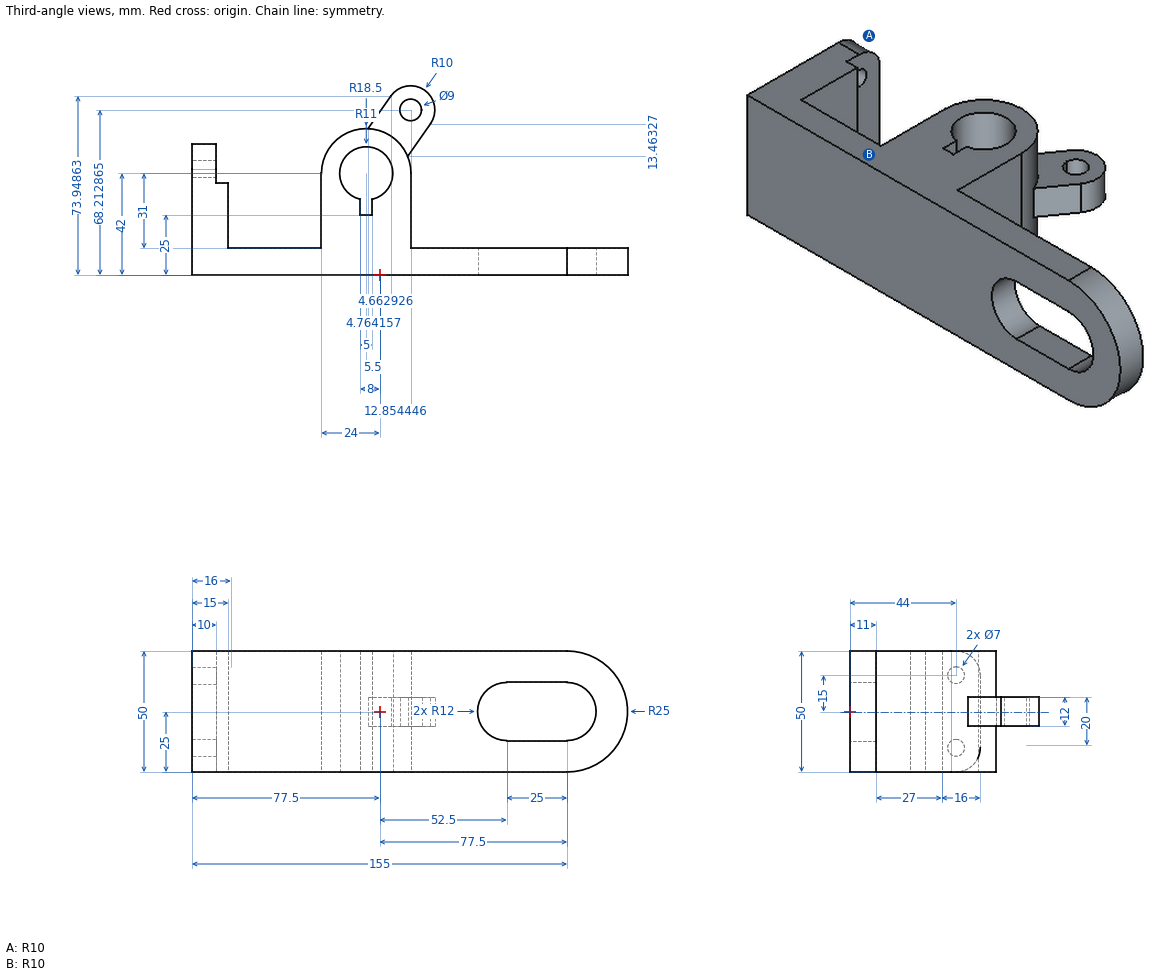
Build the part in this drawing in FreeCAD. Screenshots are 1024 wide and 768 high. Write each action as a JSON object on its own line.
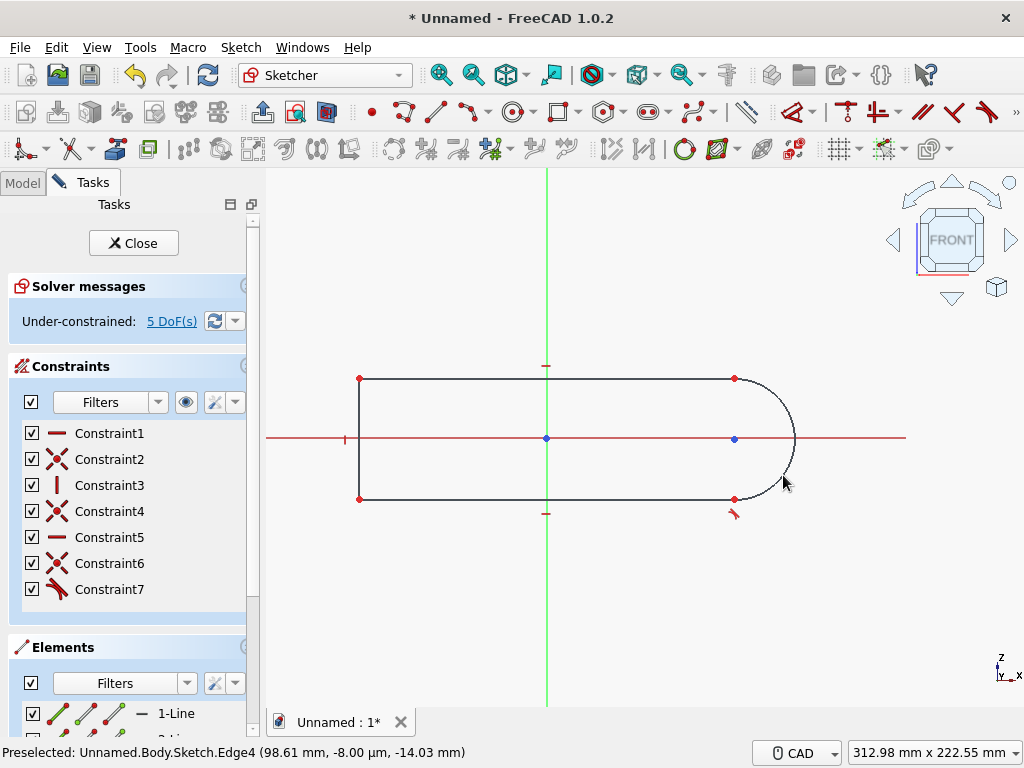
{"action": "left_click", "coordinate": [472, 379]}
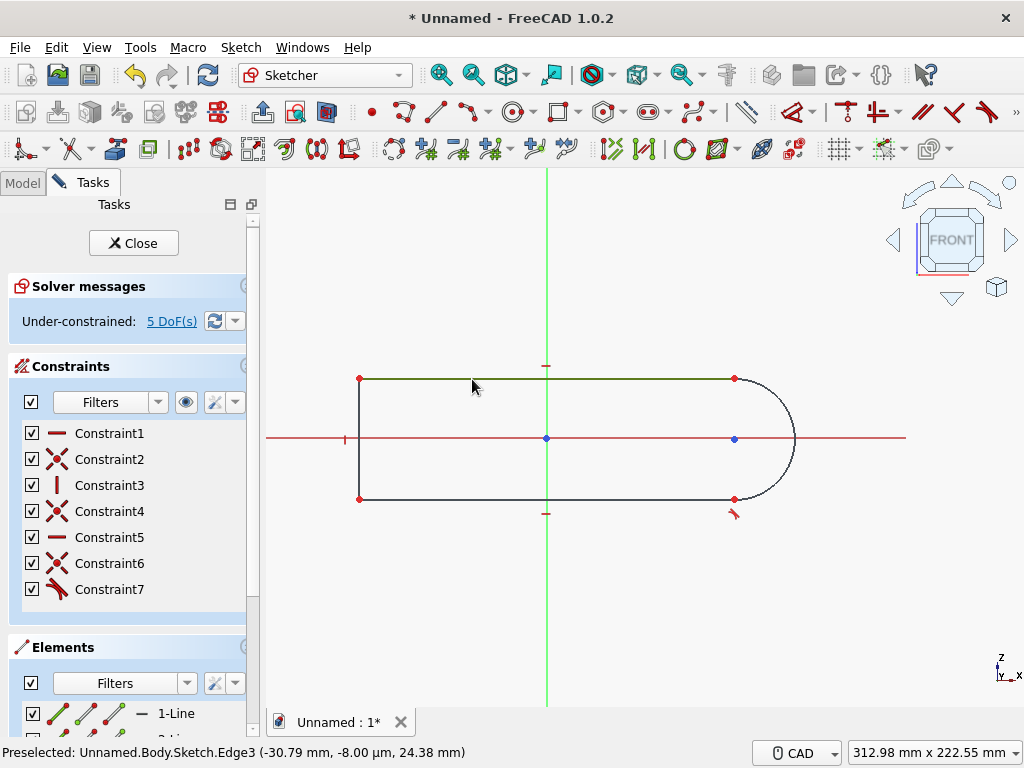
{"action": "left_click", "coordinate": [783, 475]}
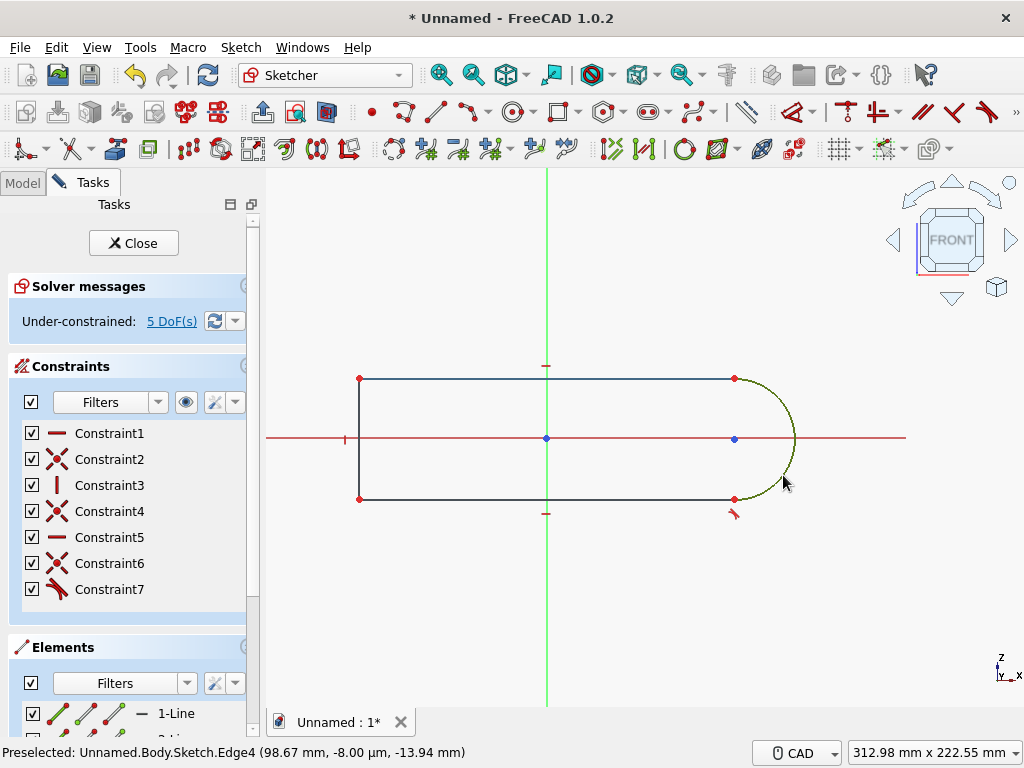
{"action": "key", "text": "t"}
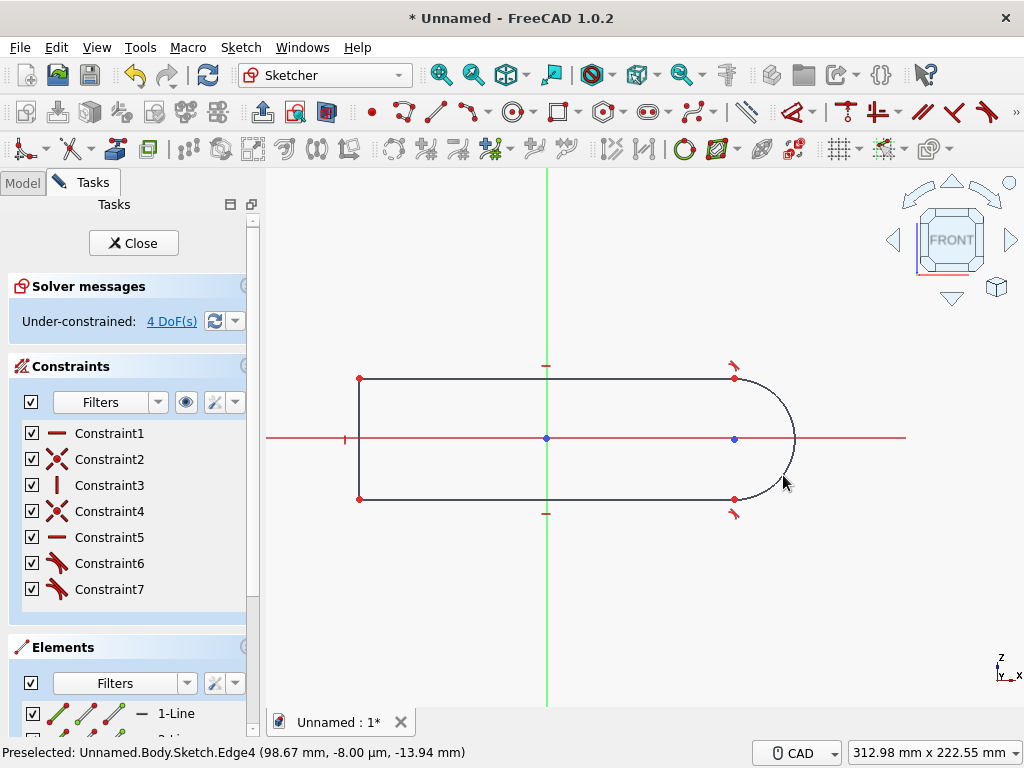
{"action": "left_click", "coordinate": [734, 439]}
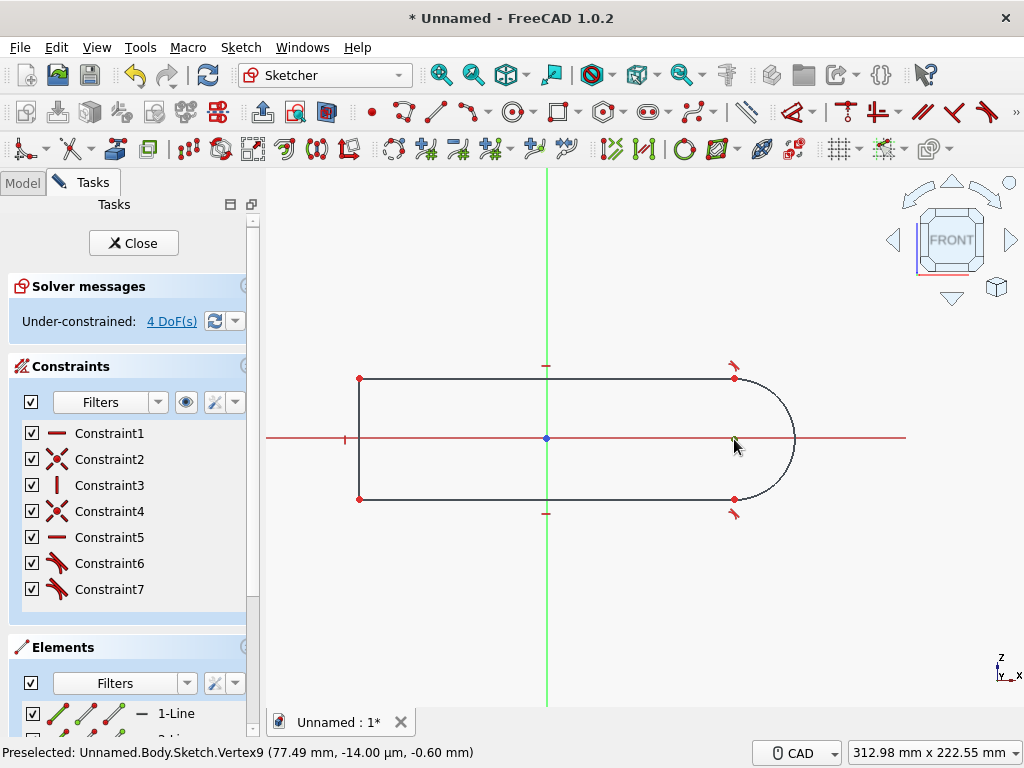
{"action": "left_click", "coordinate": [415, 438]}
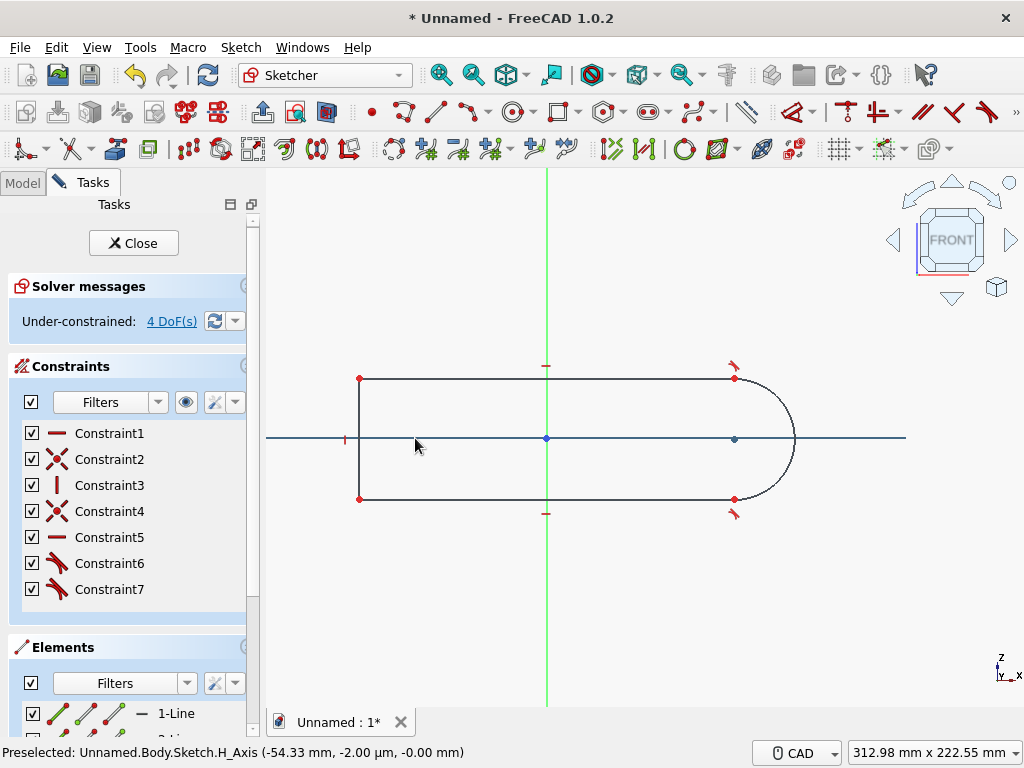
{"action": "left_click", "coordinate": [846, 112]}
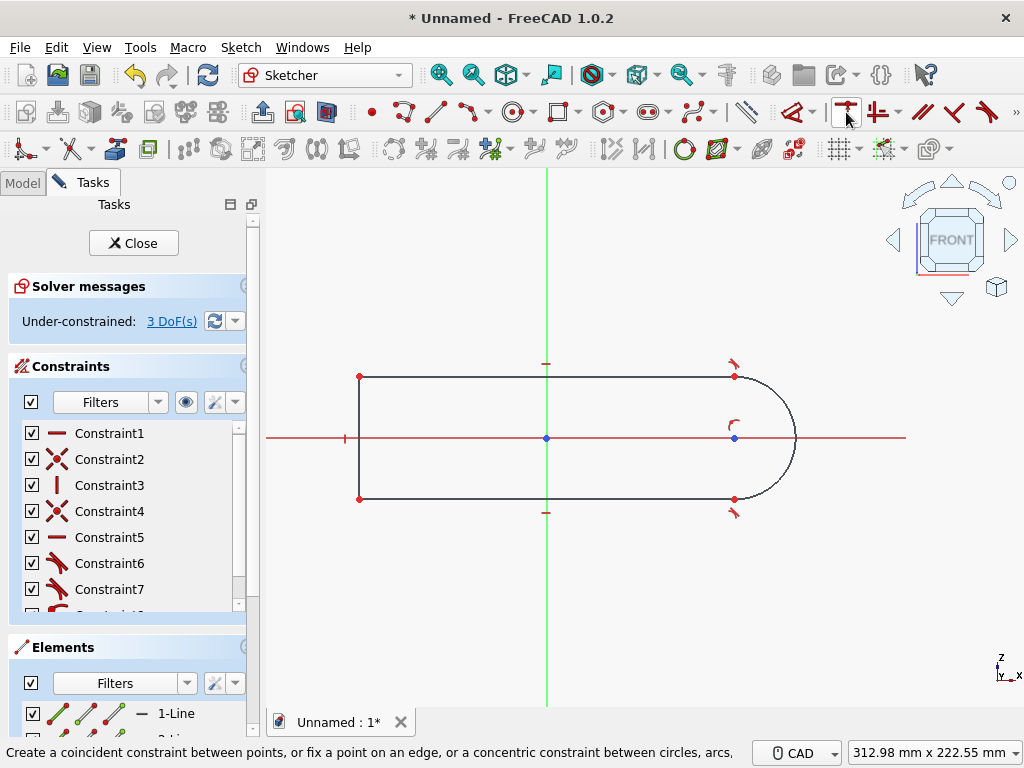
{"action": "left_click", "coordinate": [784, 474]}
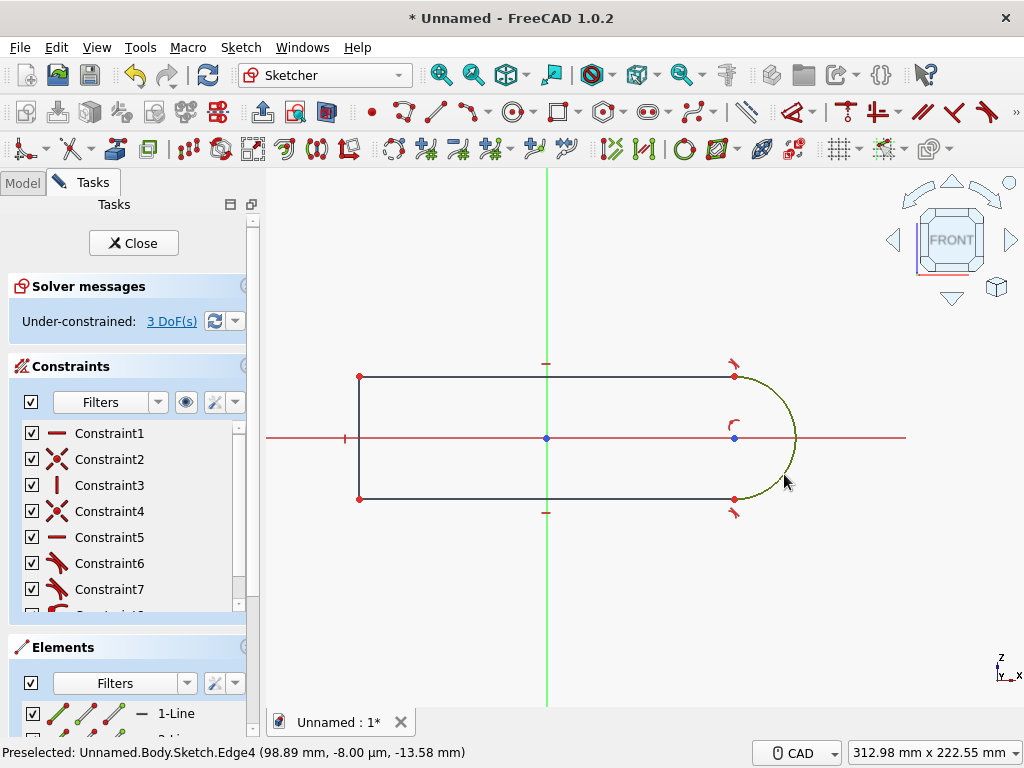
{"action": "left_click", "coordinate": [814, 112]}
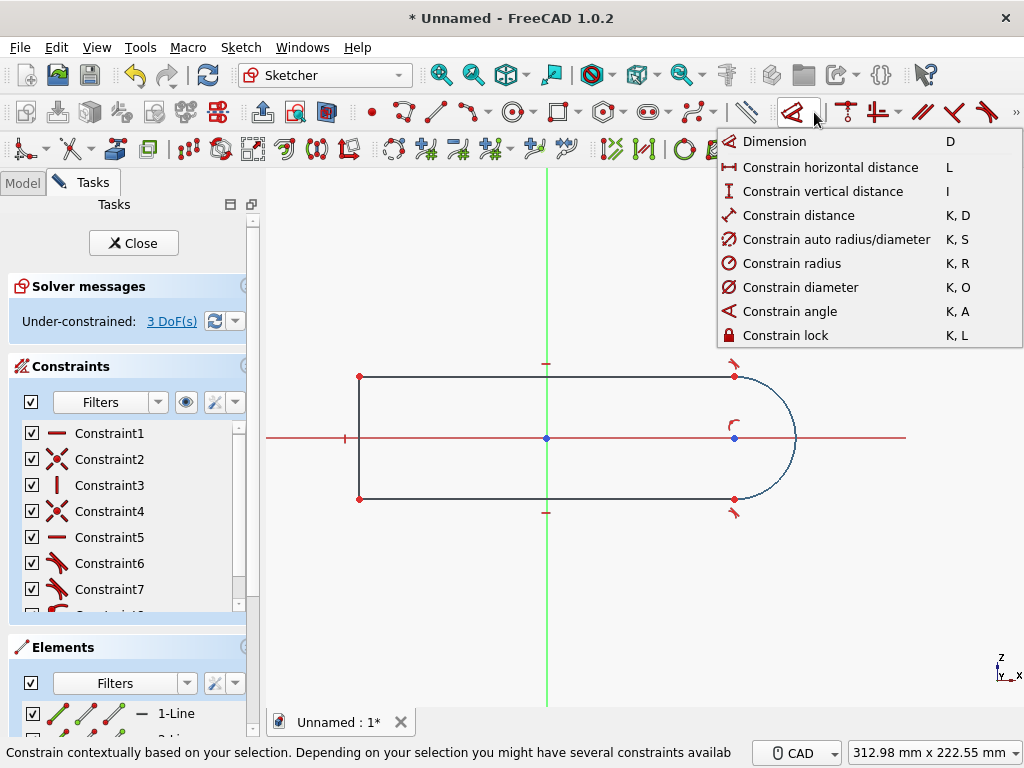
{"action": "left_click", "coordinate": [870, 263]}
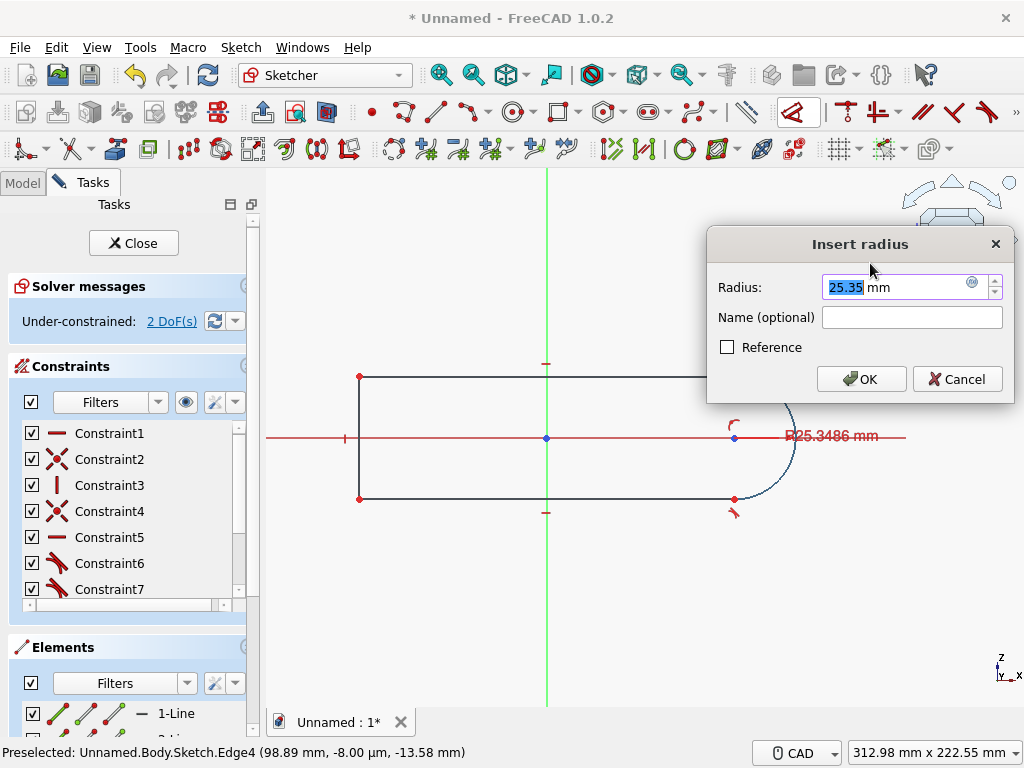
{"action": "type", "text": "25"}
{"action": "key", "text": "Return"}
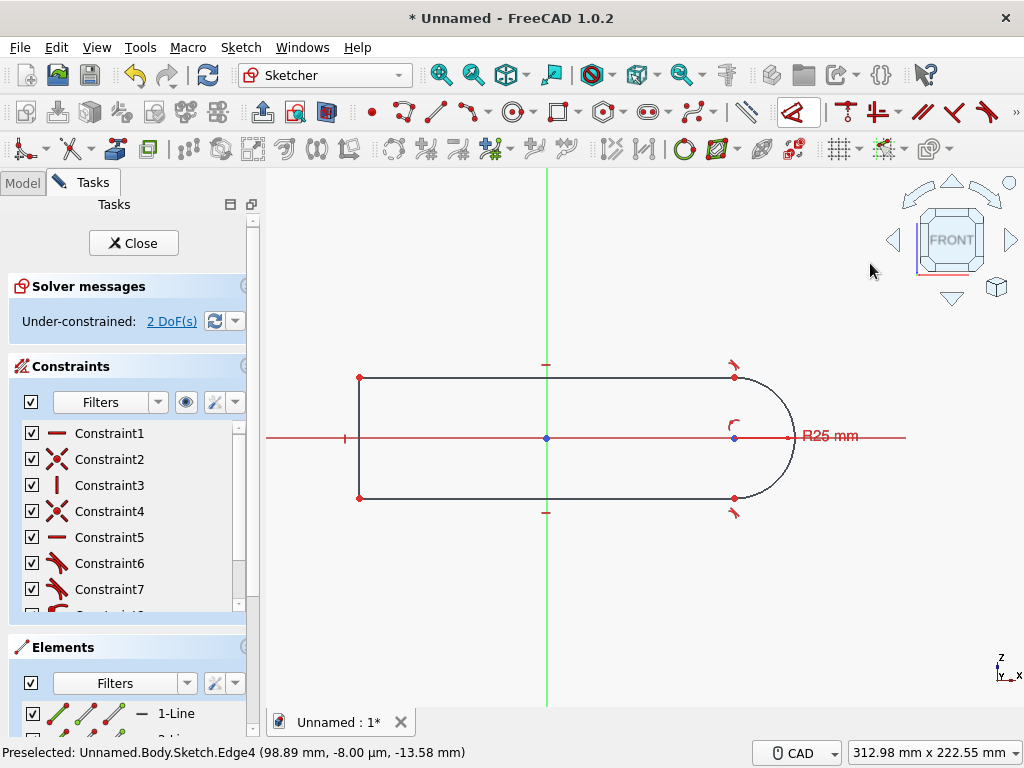
{"action": "left_click", "coordinate": [622, 499]}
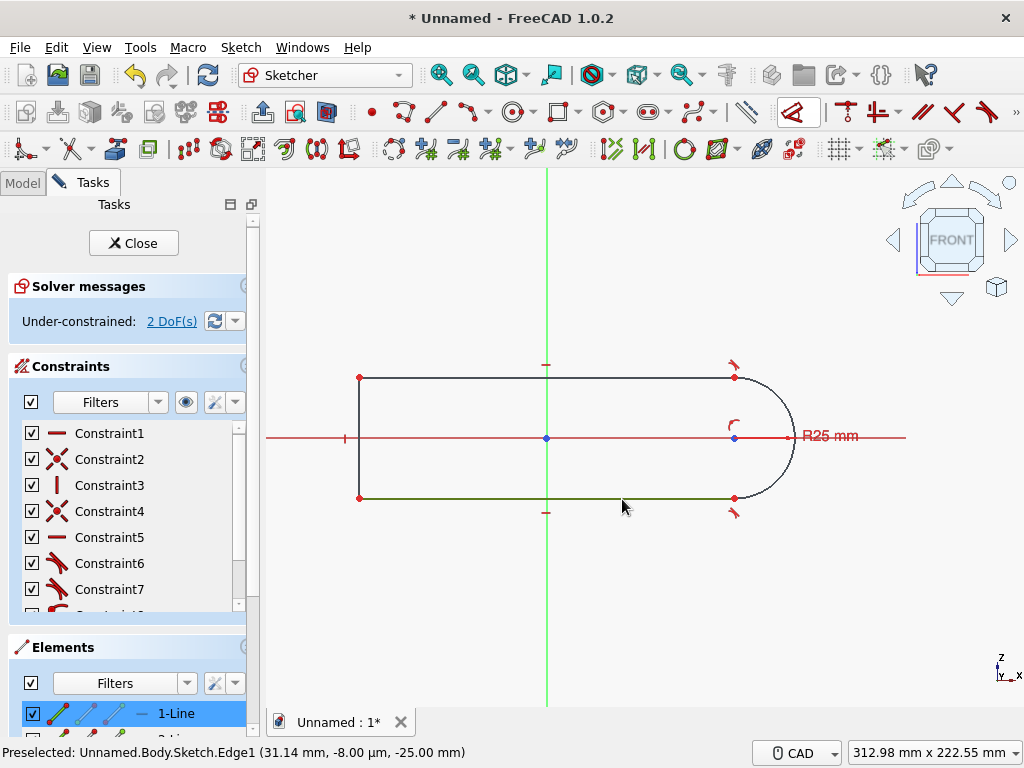
{"action": "key", "text": "l"}